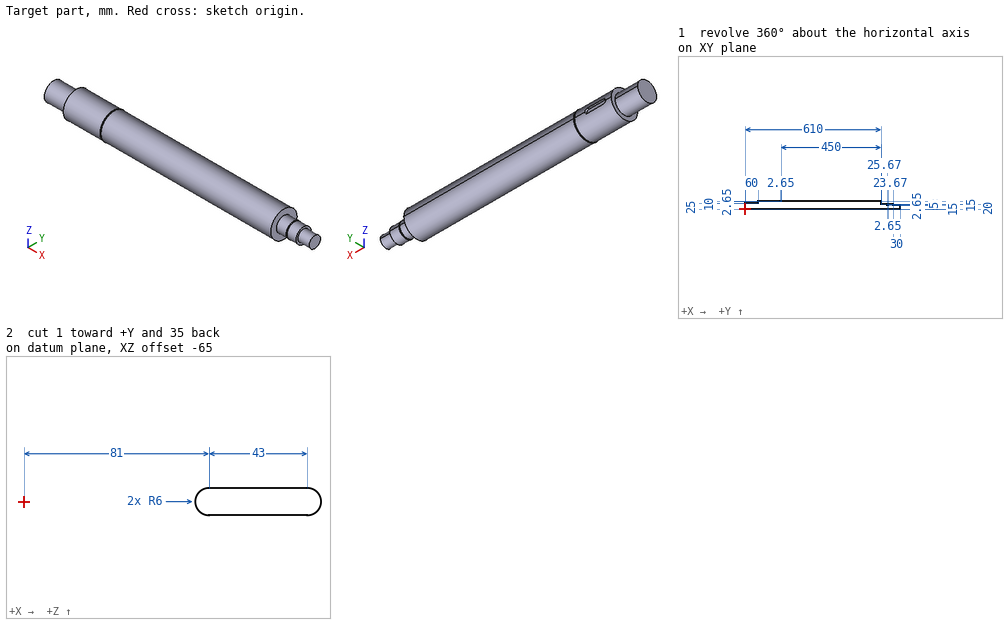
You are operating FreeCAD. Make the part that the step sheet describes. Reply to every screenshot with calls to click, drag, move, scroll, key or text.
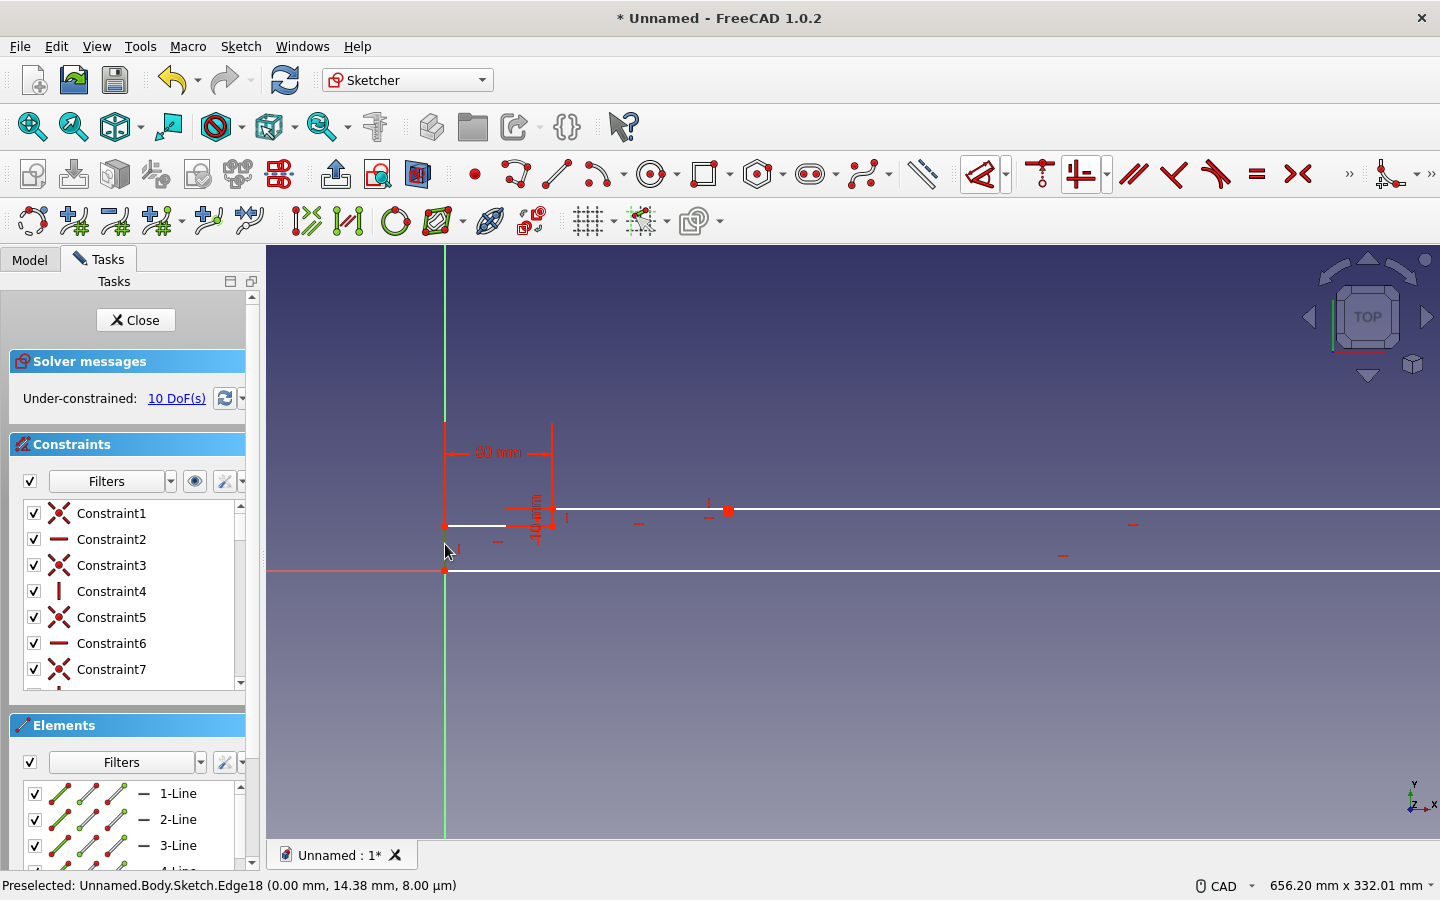
click(1006, 174)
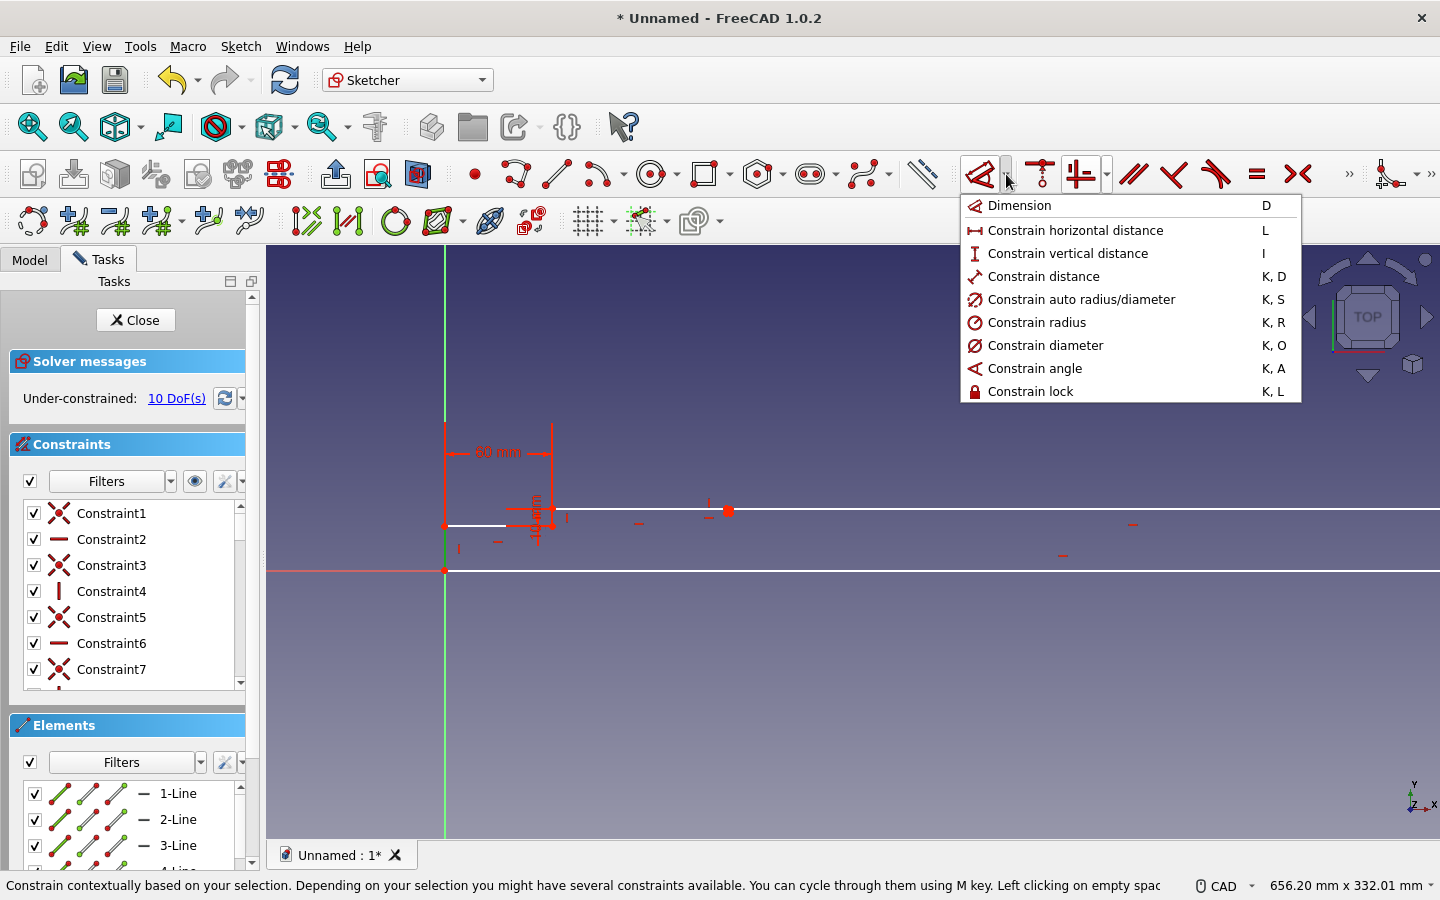
click(1131, 254)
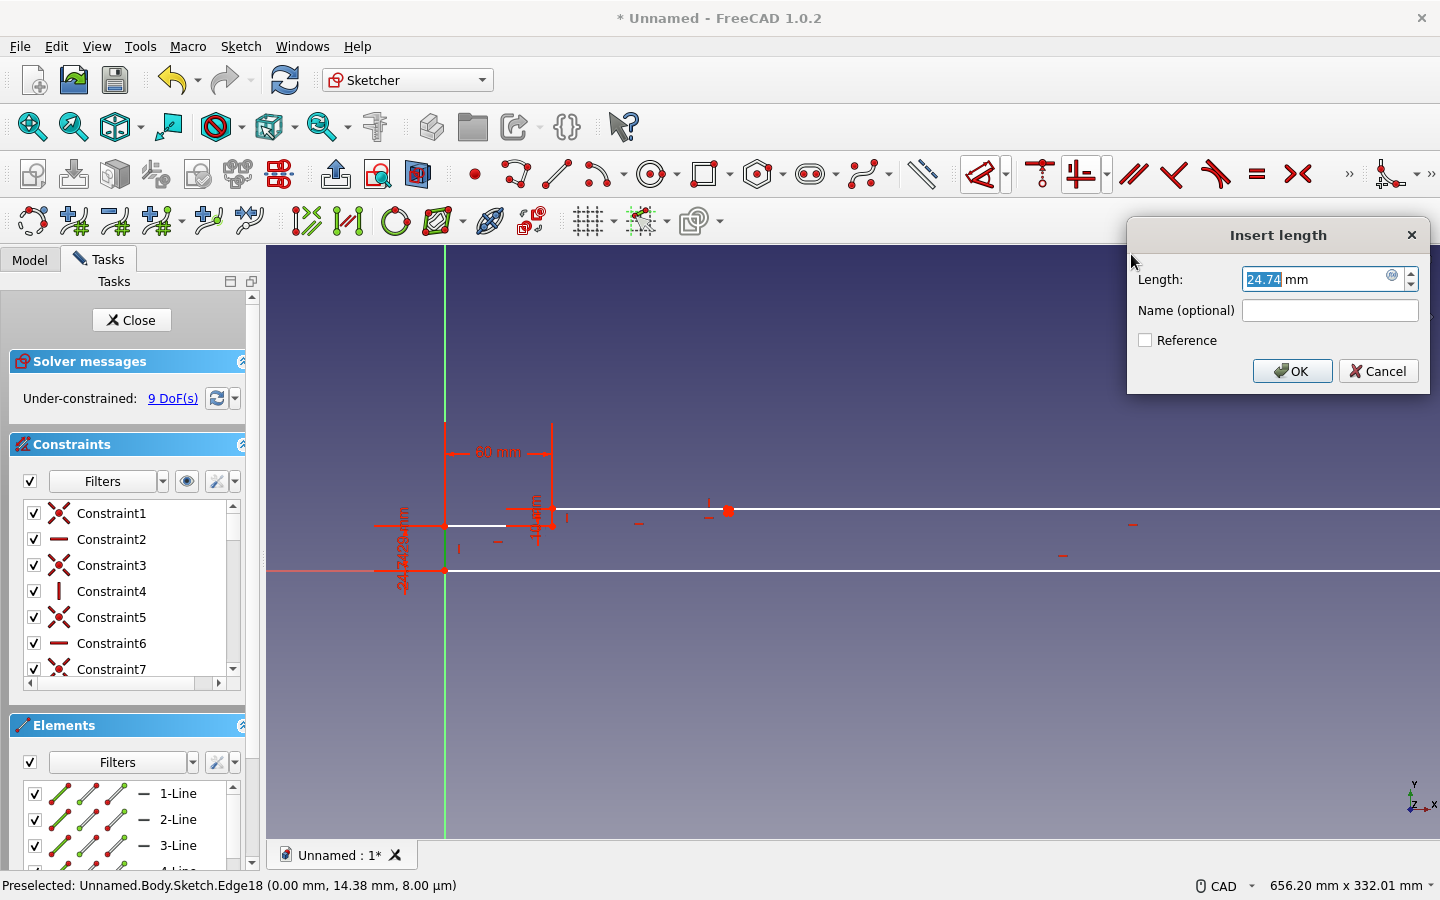
text(25)
key(Return)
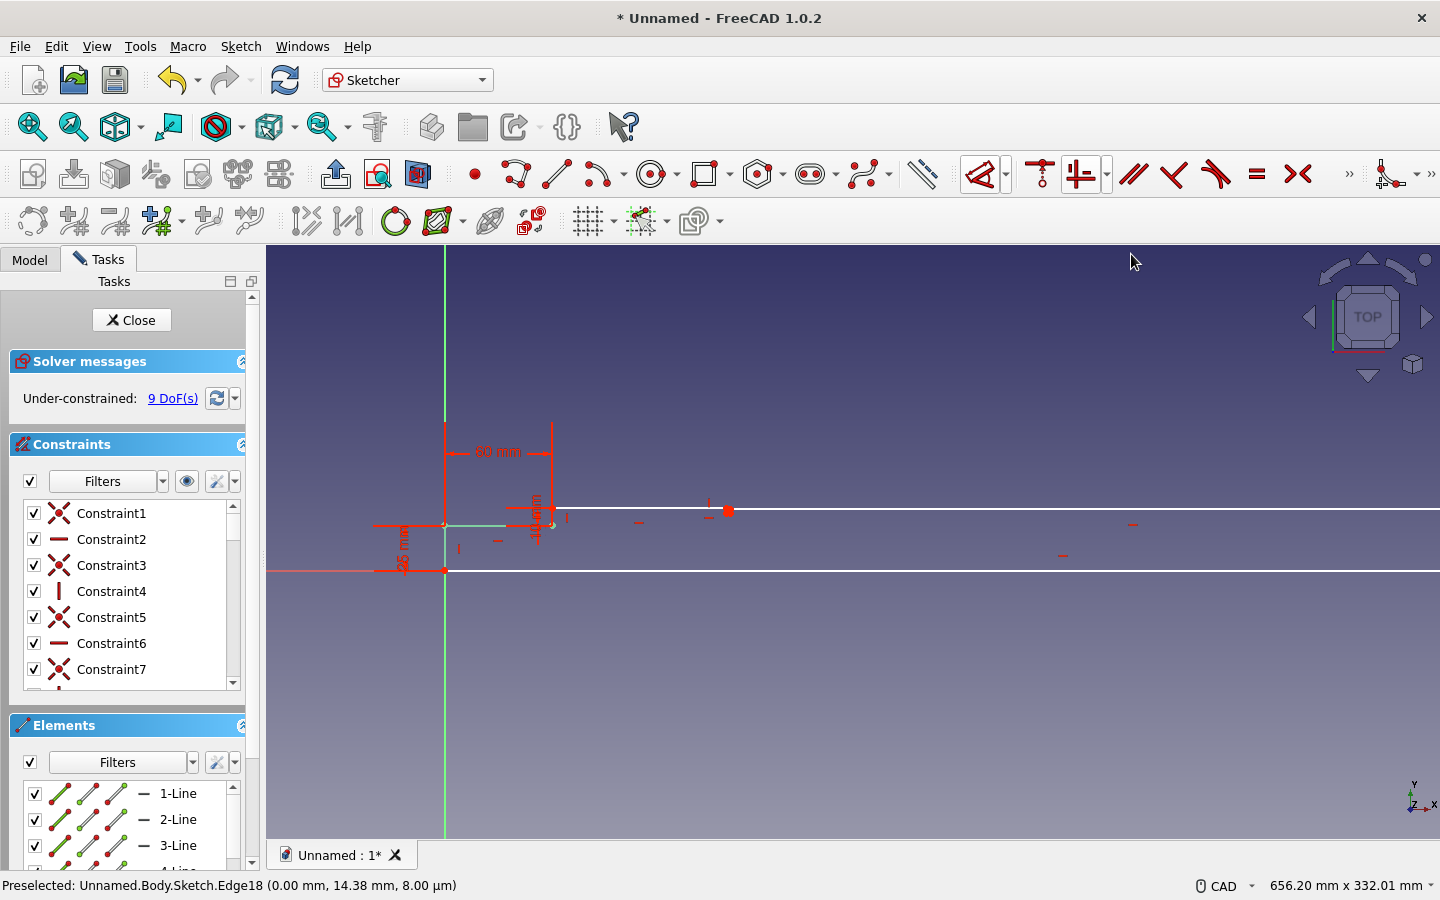
click(973, 509)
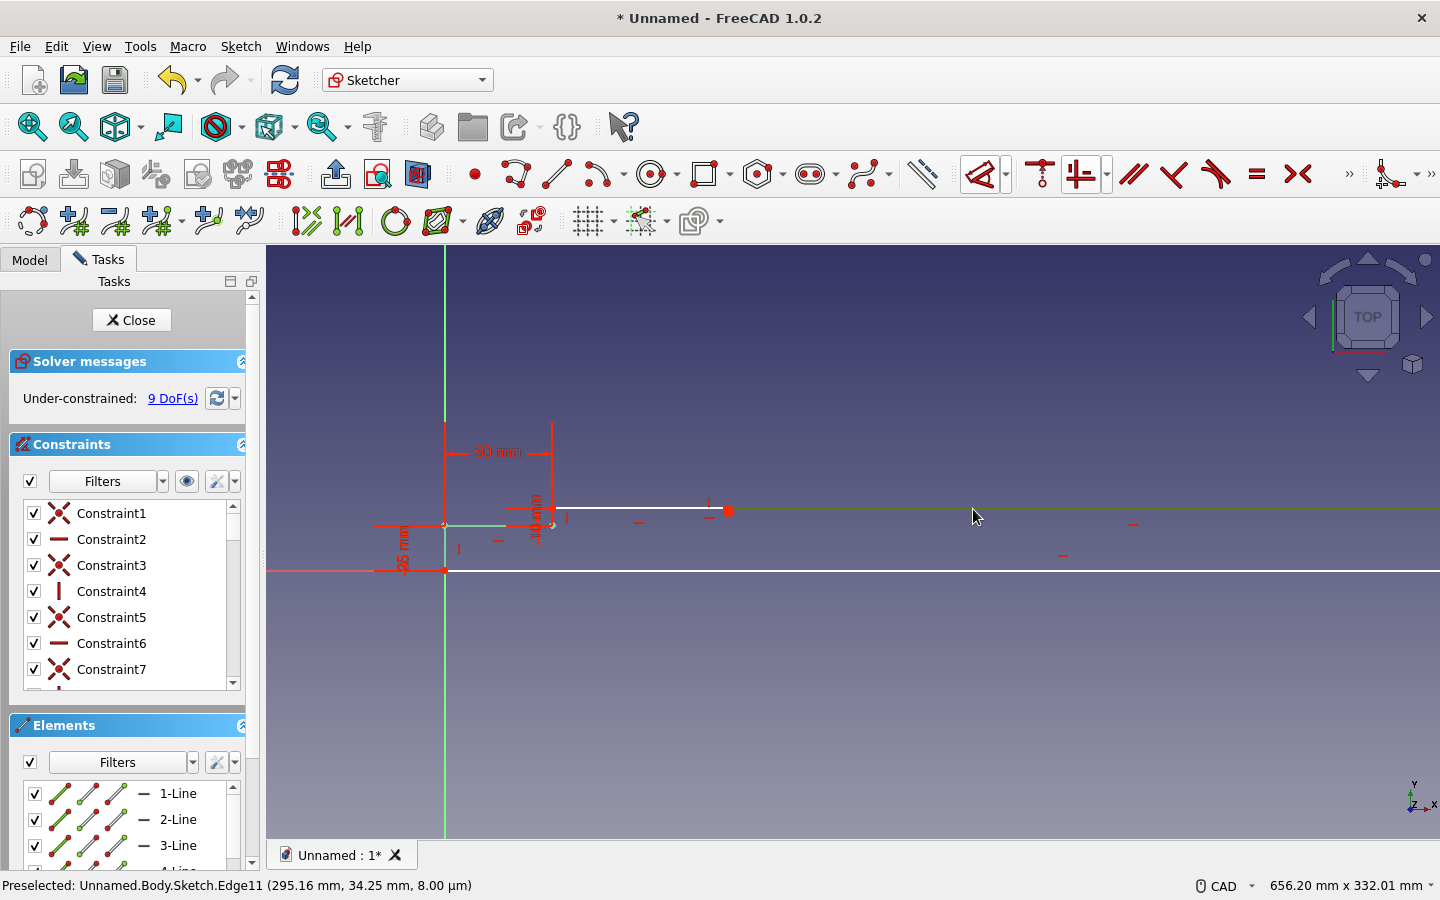
key(l)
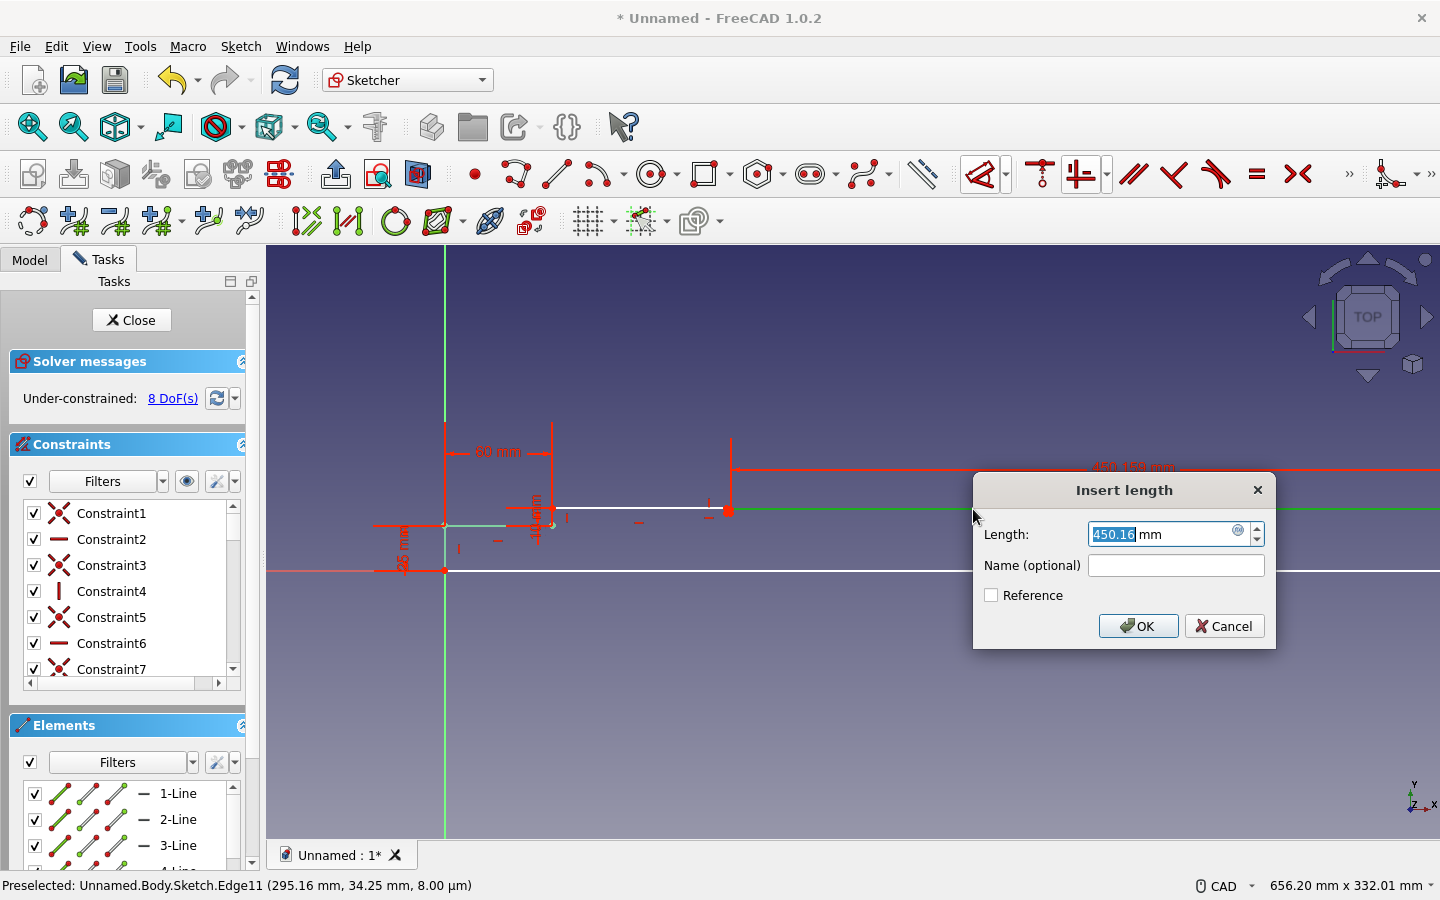
text(450)
key(Return)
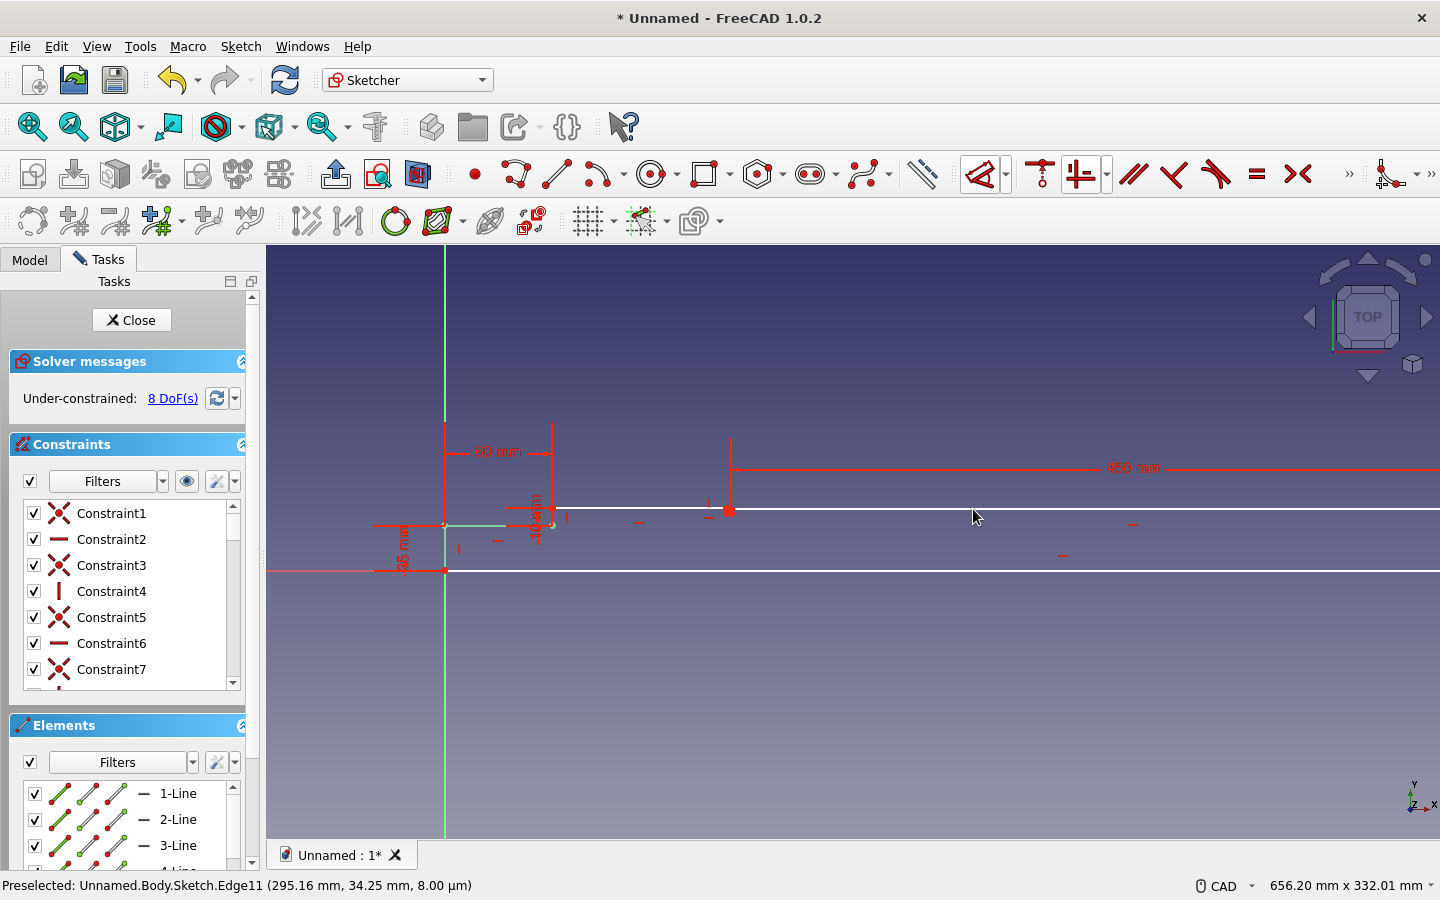
scroll(445, 545, down, 3)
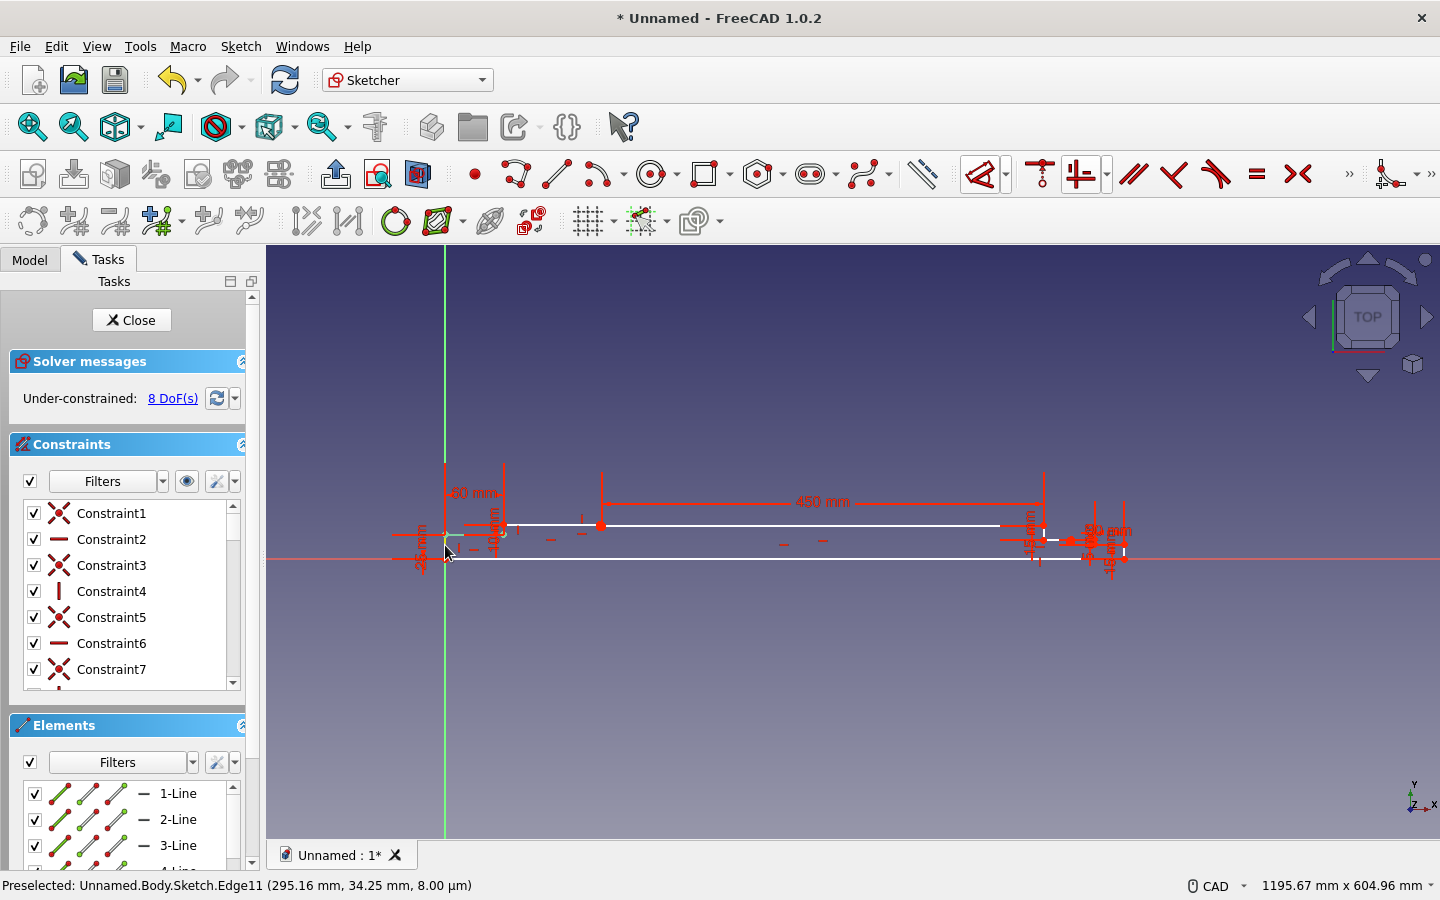
scroll(1069, 540, up, 9)